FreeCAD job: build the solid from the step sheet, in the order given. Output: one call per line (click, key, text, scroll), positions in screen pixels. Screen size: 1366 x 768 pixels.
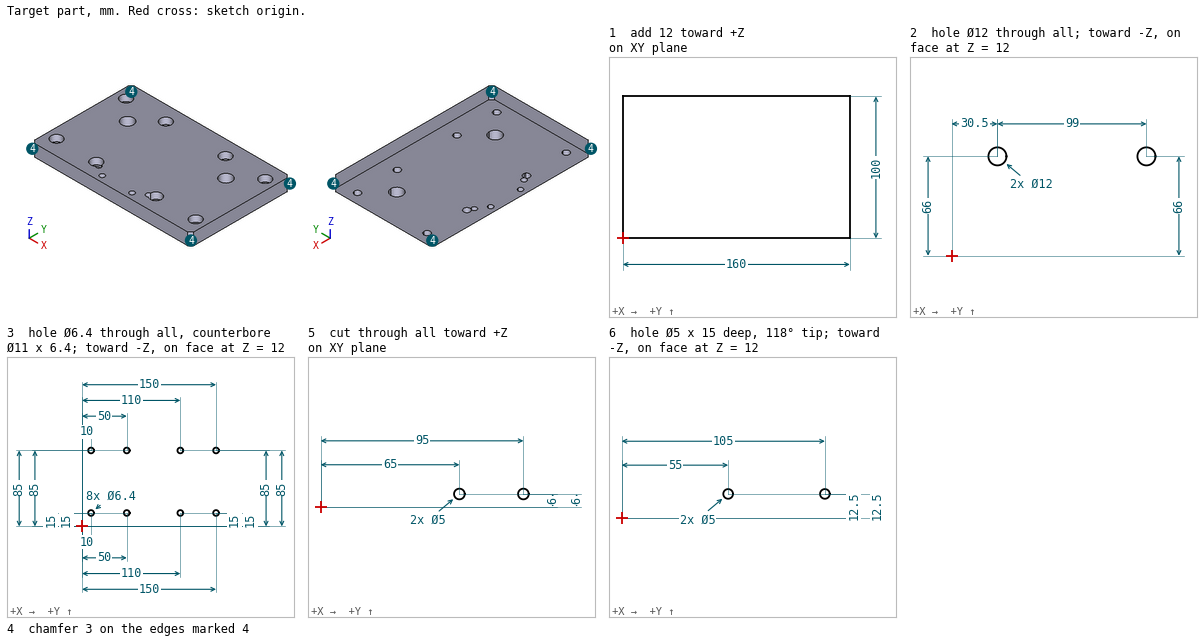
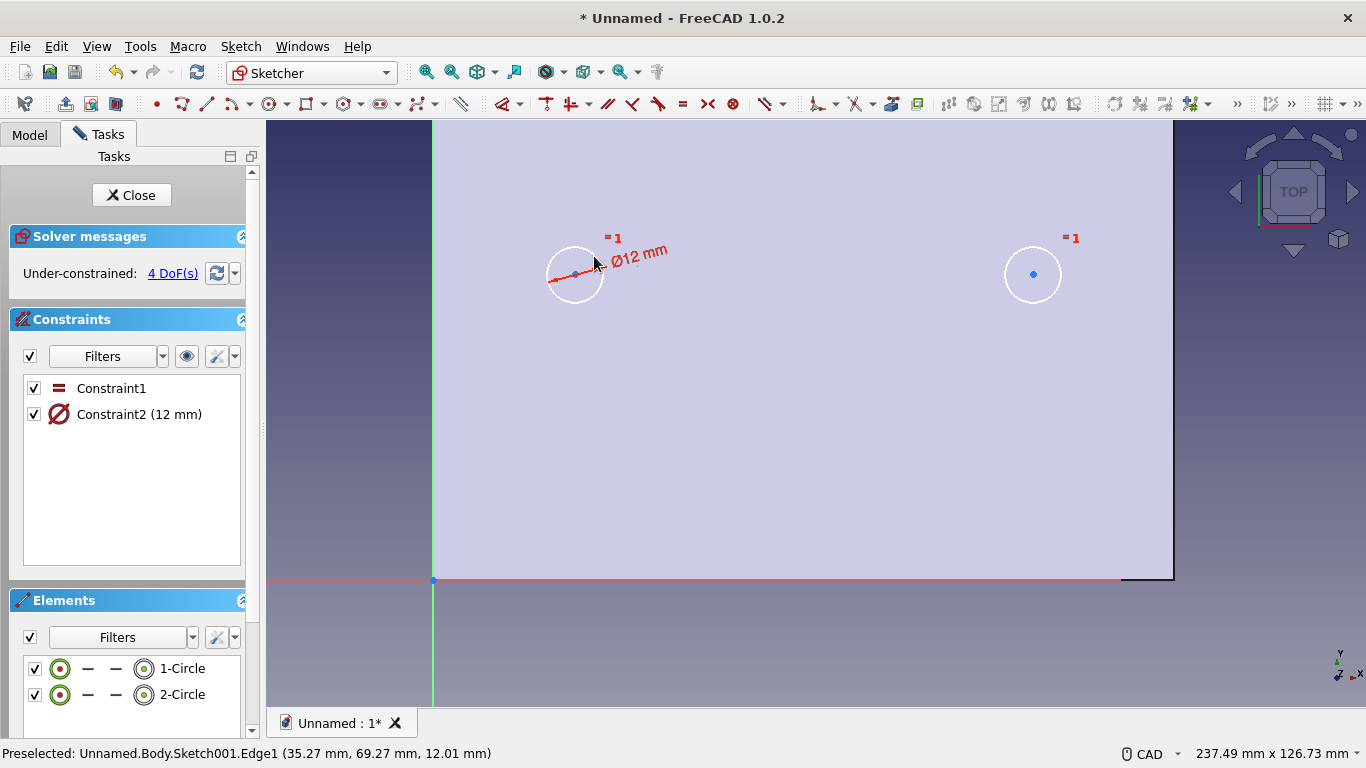
click(575, 275)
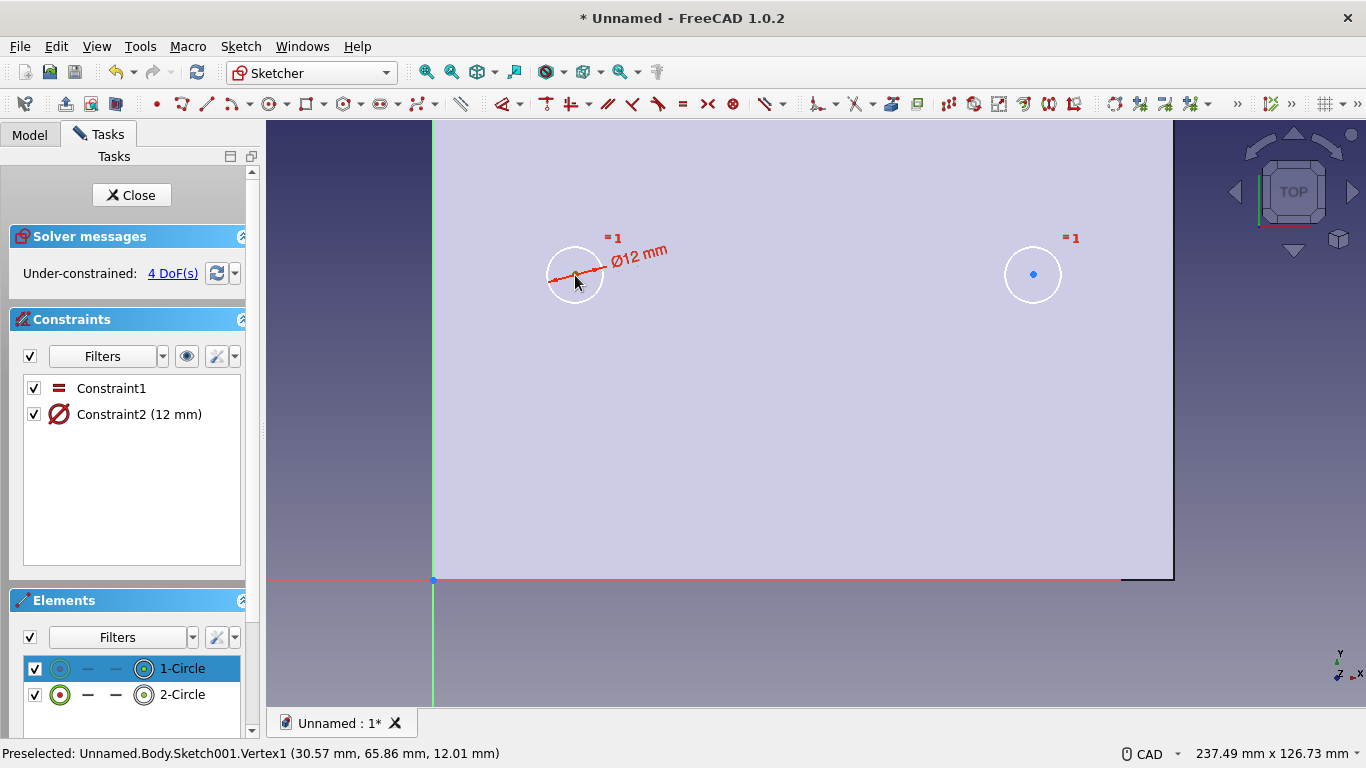
key(i)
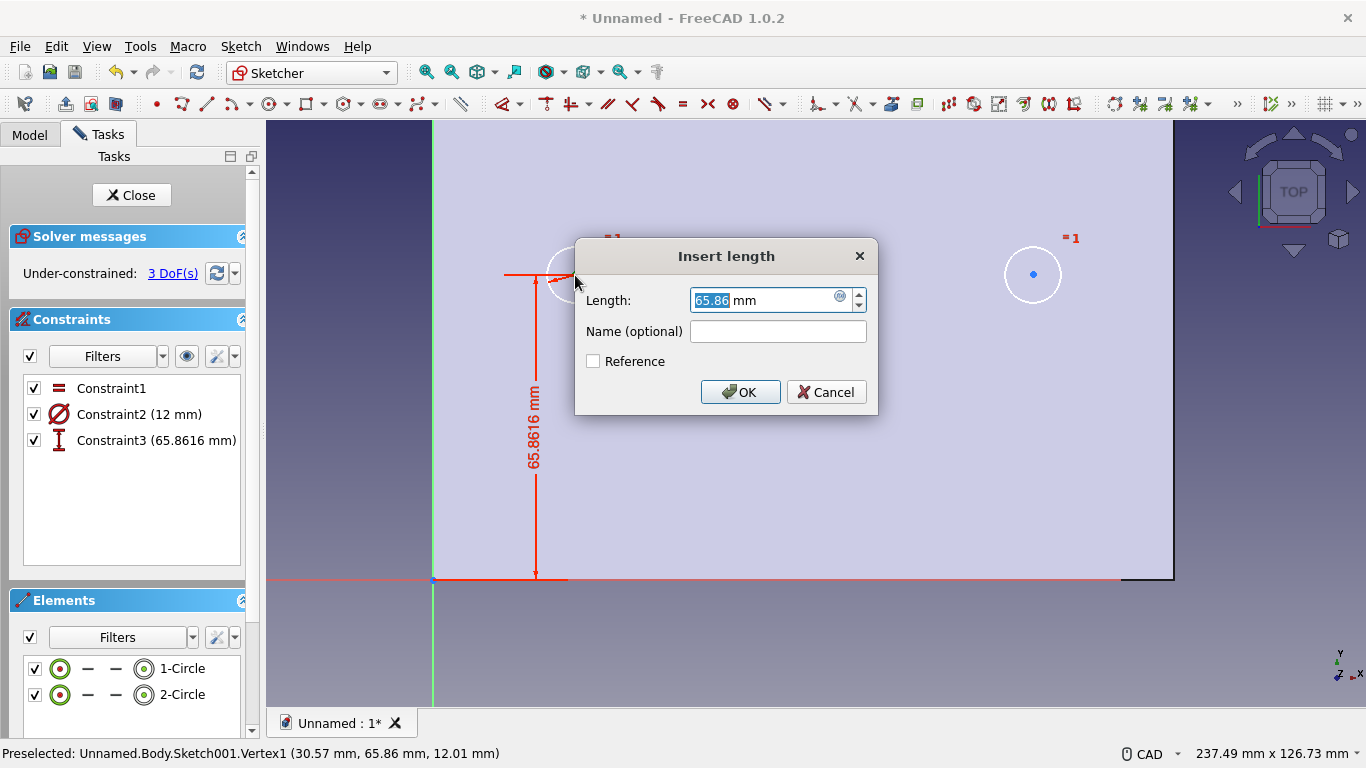
text(66)
key(Return)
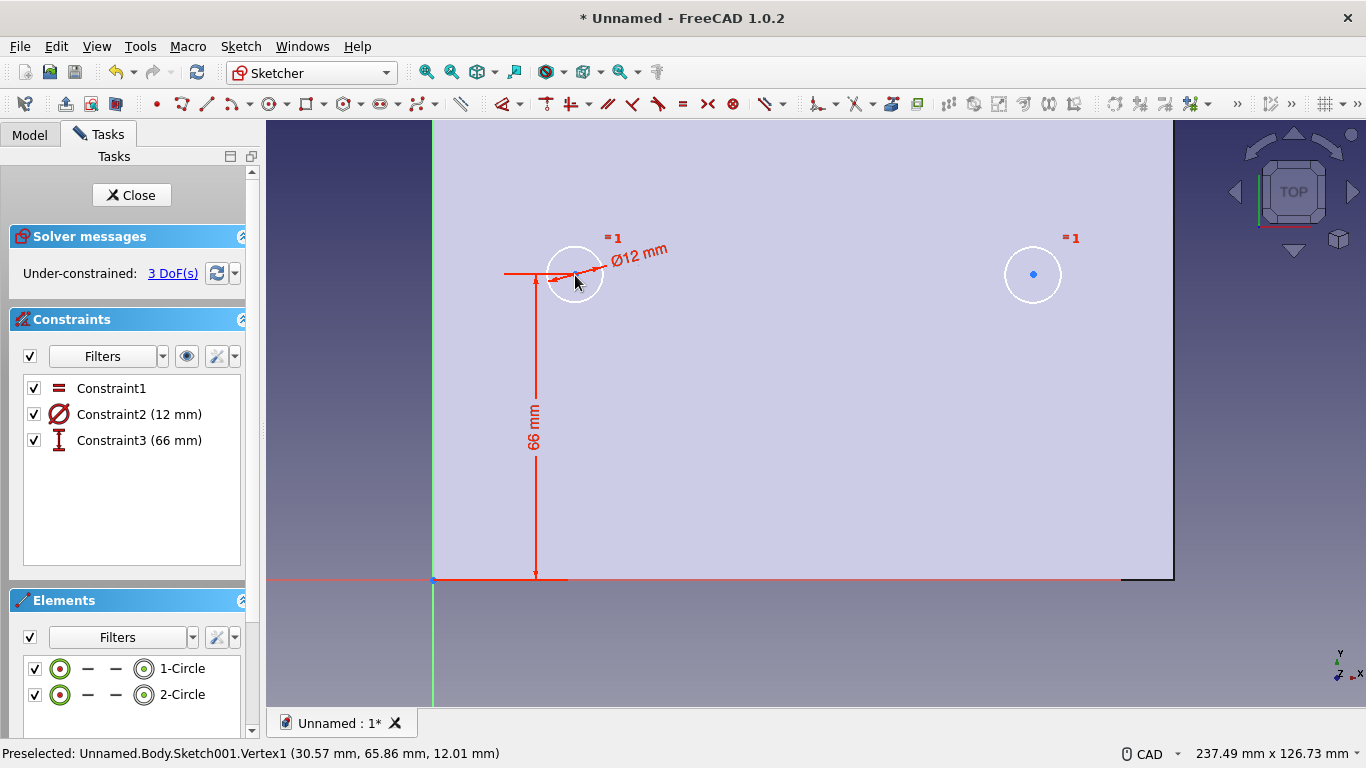
click(1033, 275)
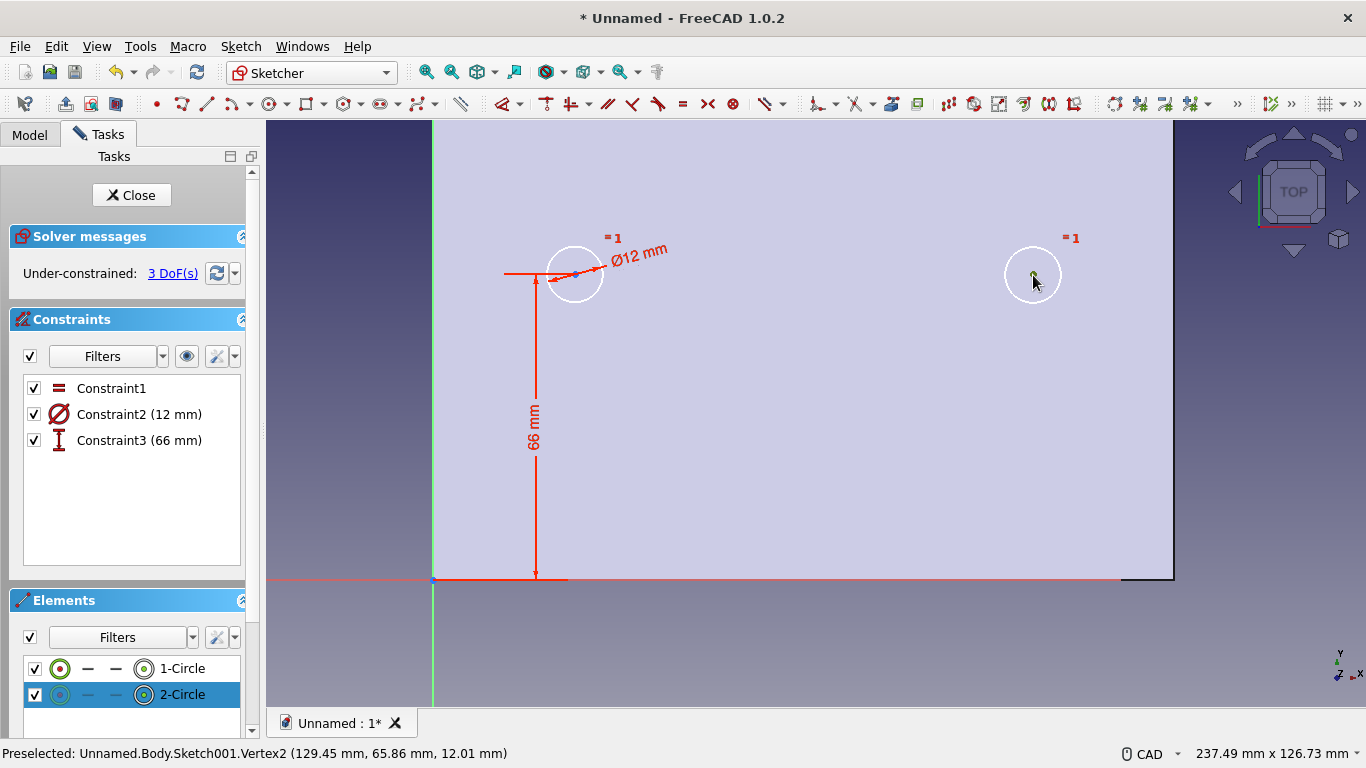
key(i)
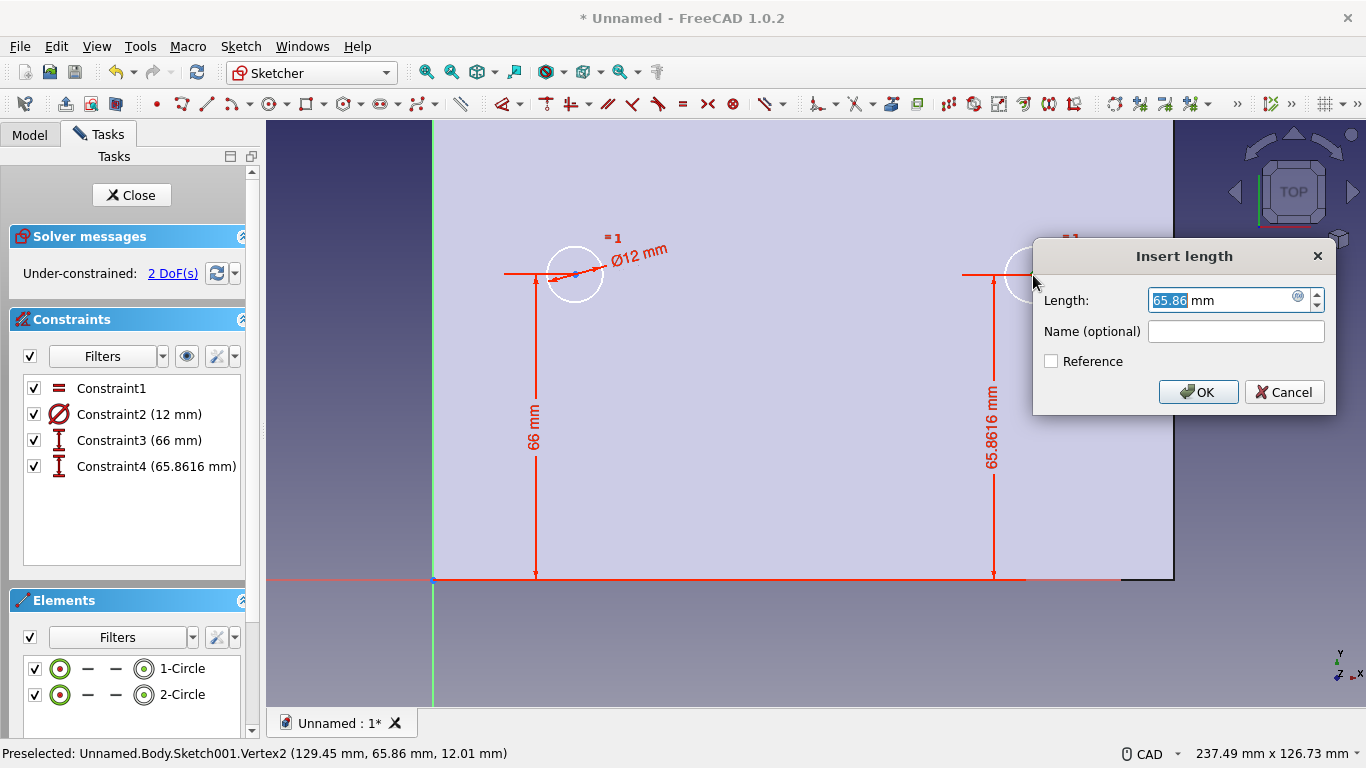
text(66)
key(Return)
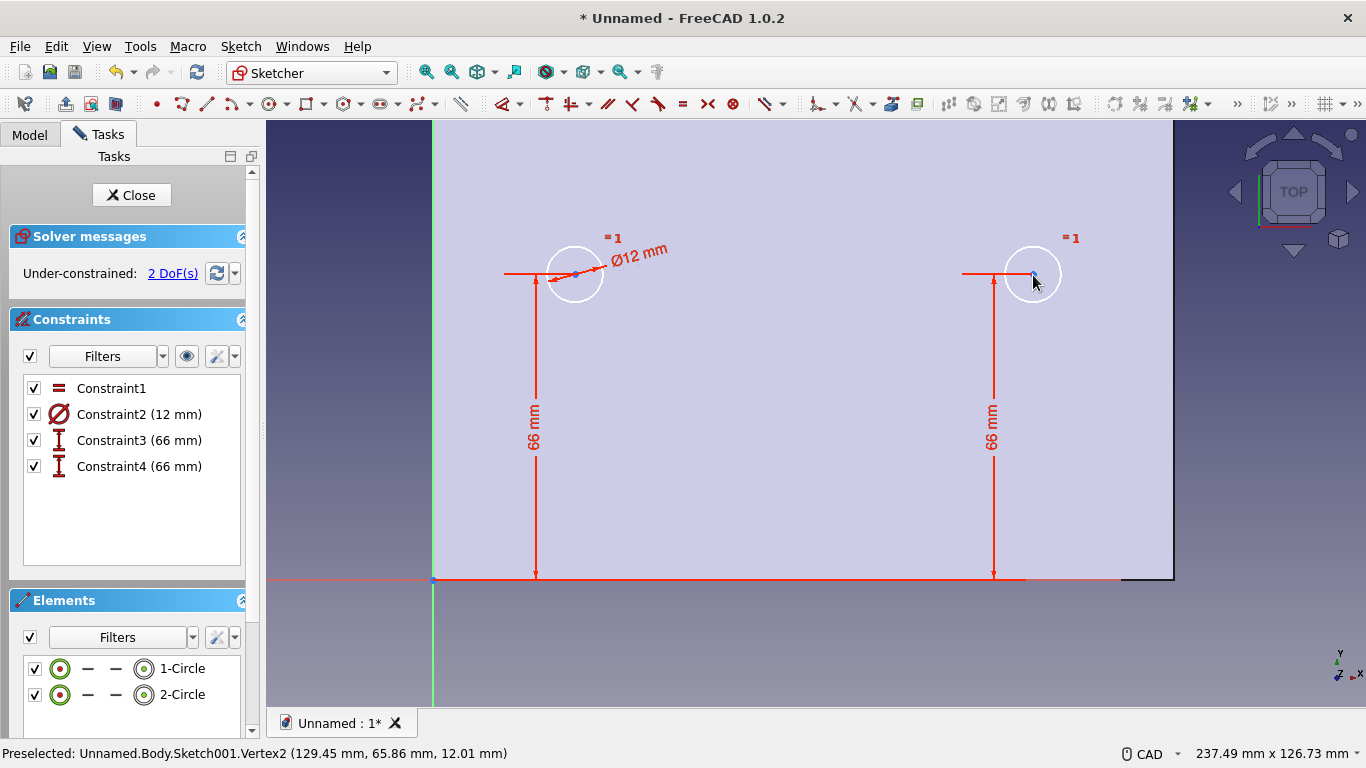
click(575, 274)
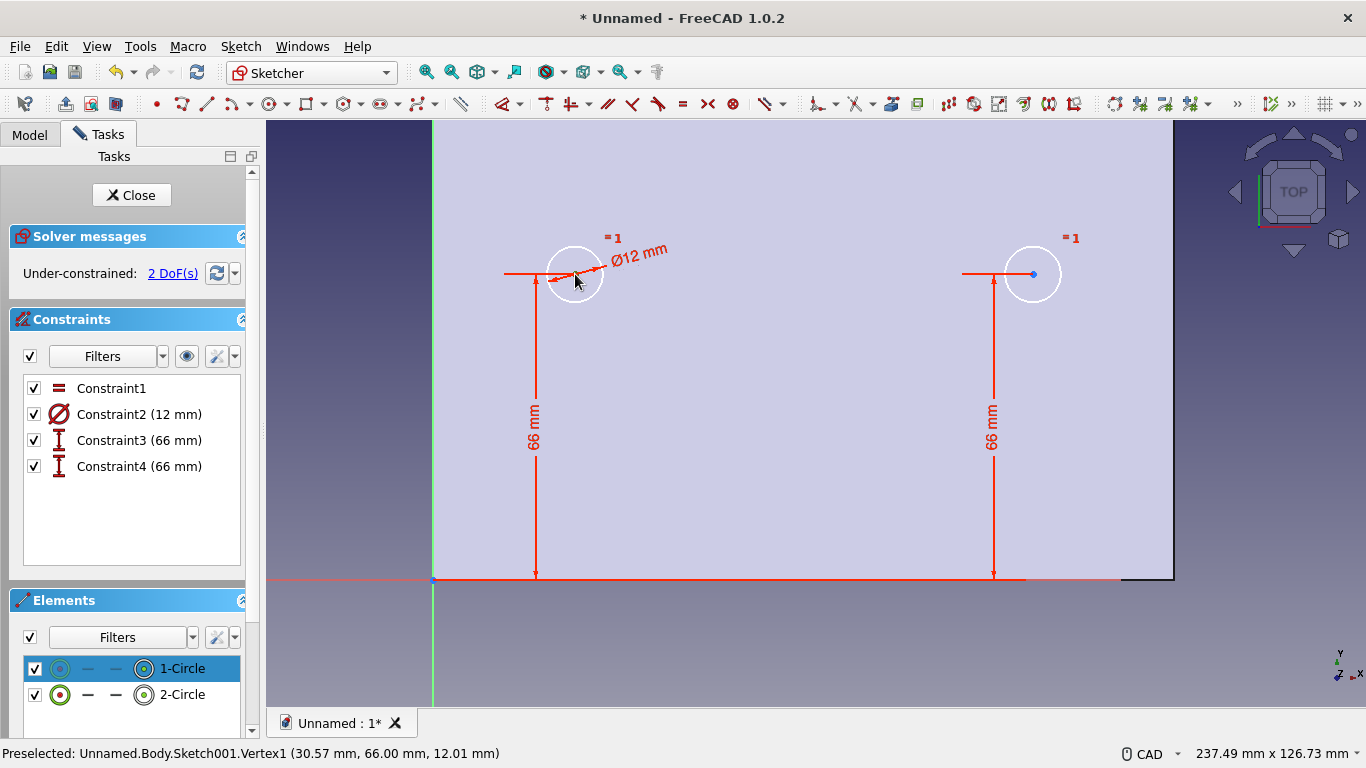
click(1033, 274)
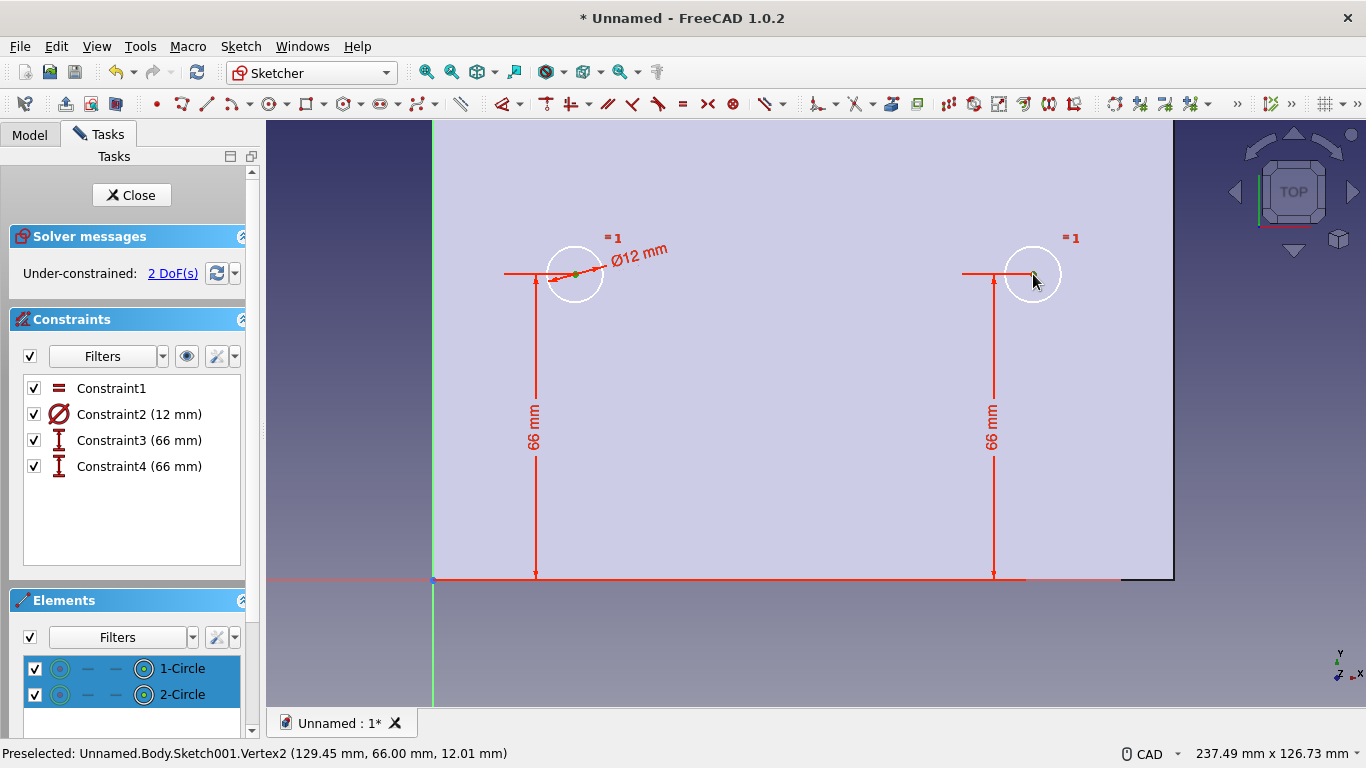
key(l)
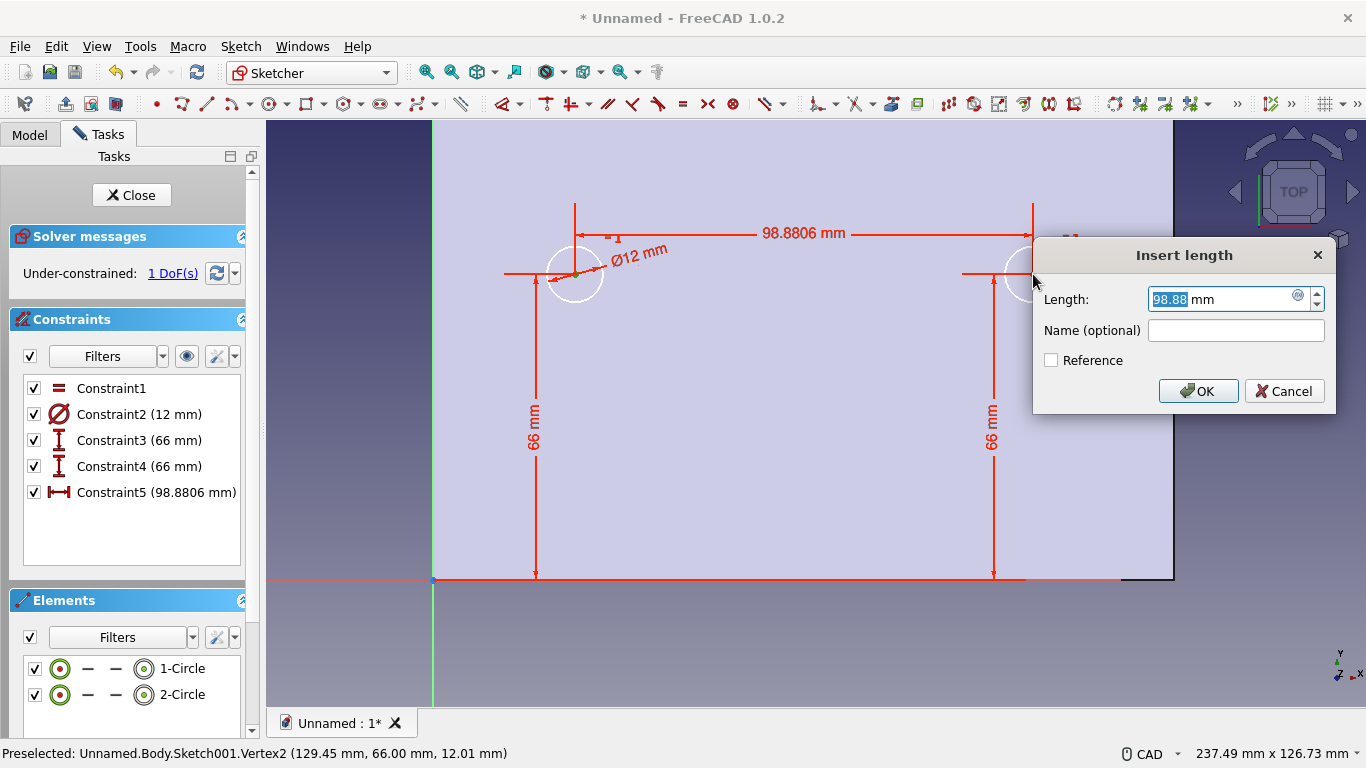
text(99)
key(Return)